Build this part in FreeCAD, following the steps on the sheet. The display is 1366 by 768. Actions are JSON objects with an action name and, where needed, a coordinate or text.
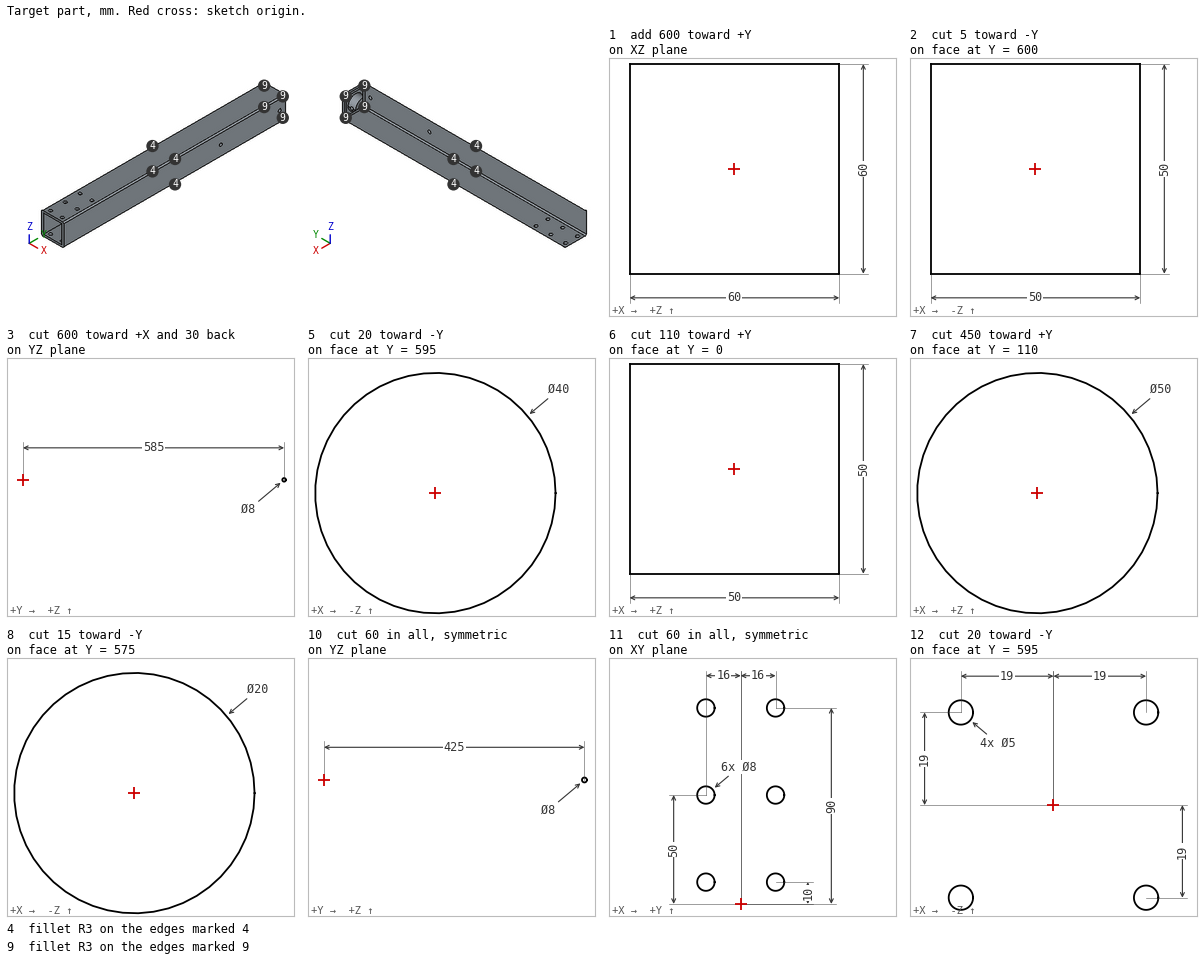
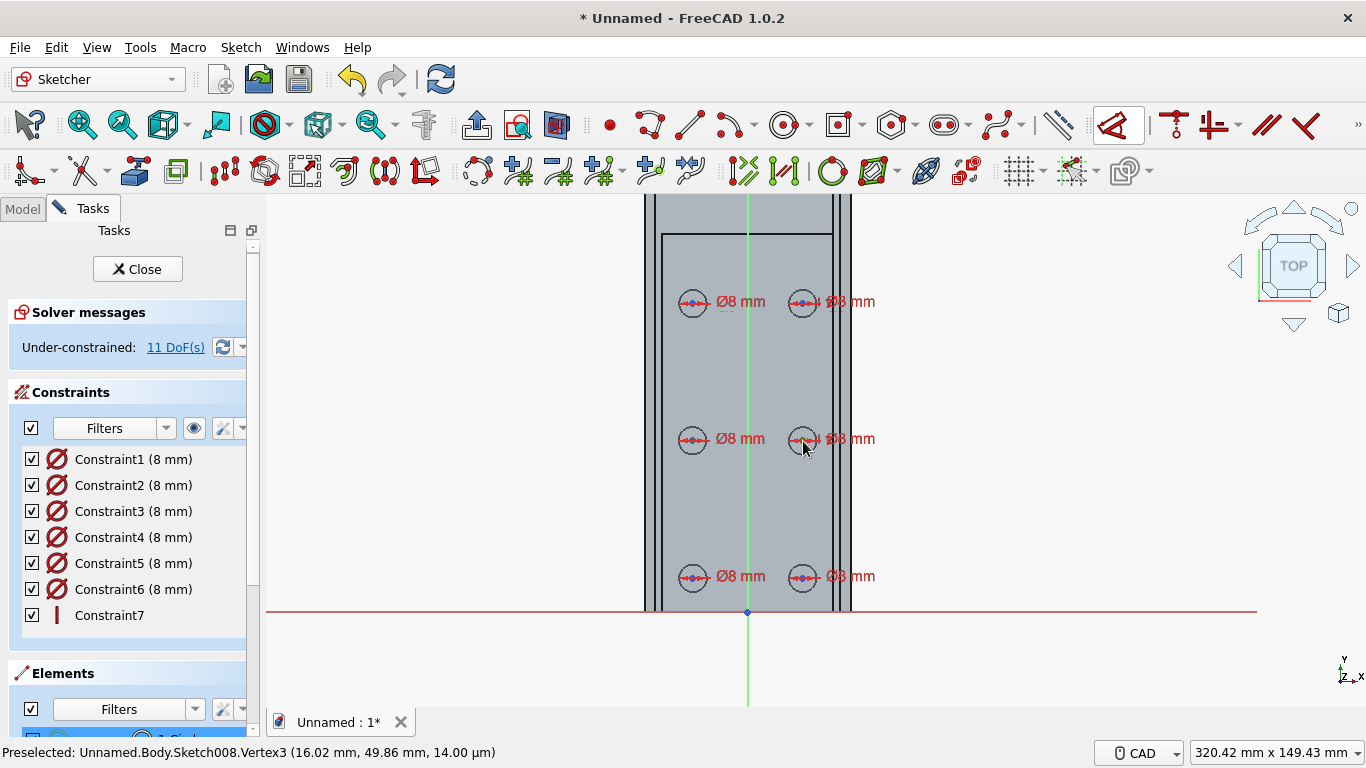
{"action": "key", "text": "h"}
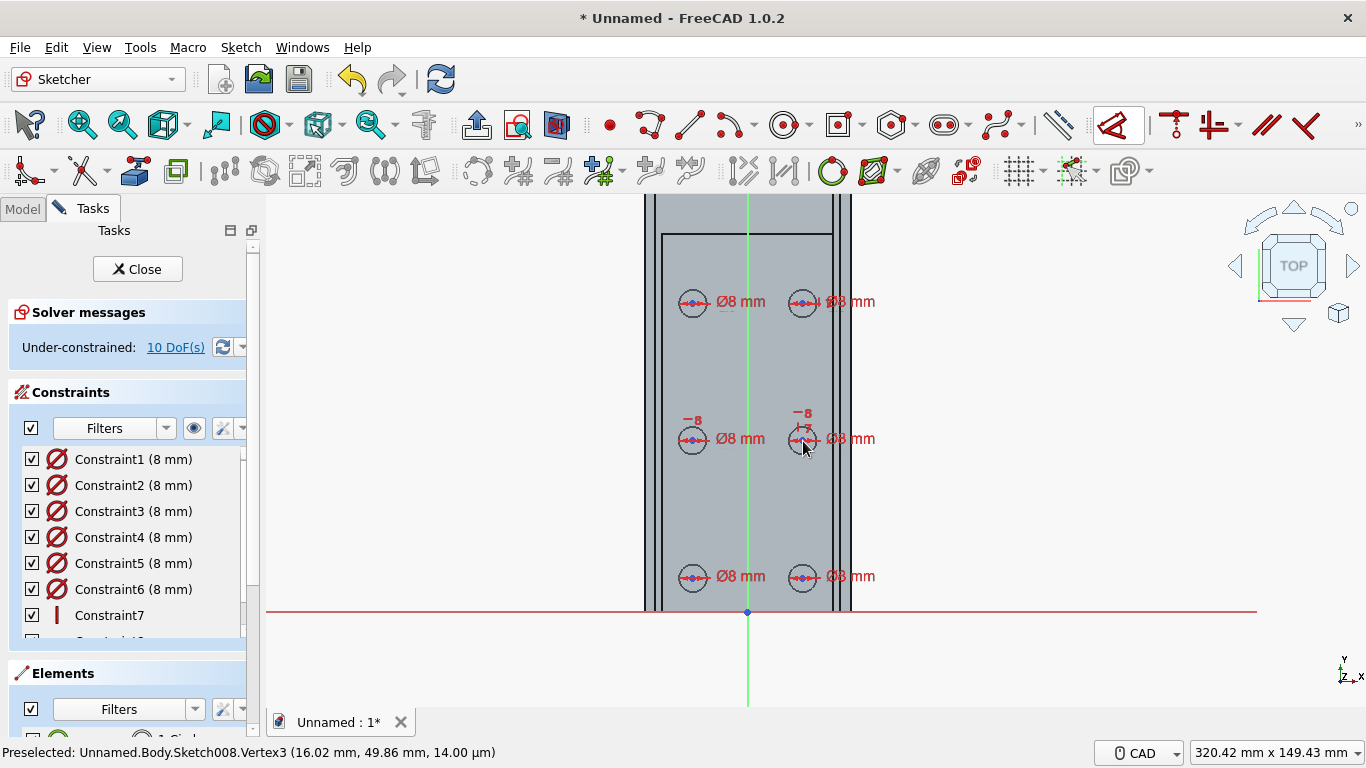
{"action": "left_click", "coordinate": [692, 441]}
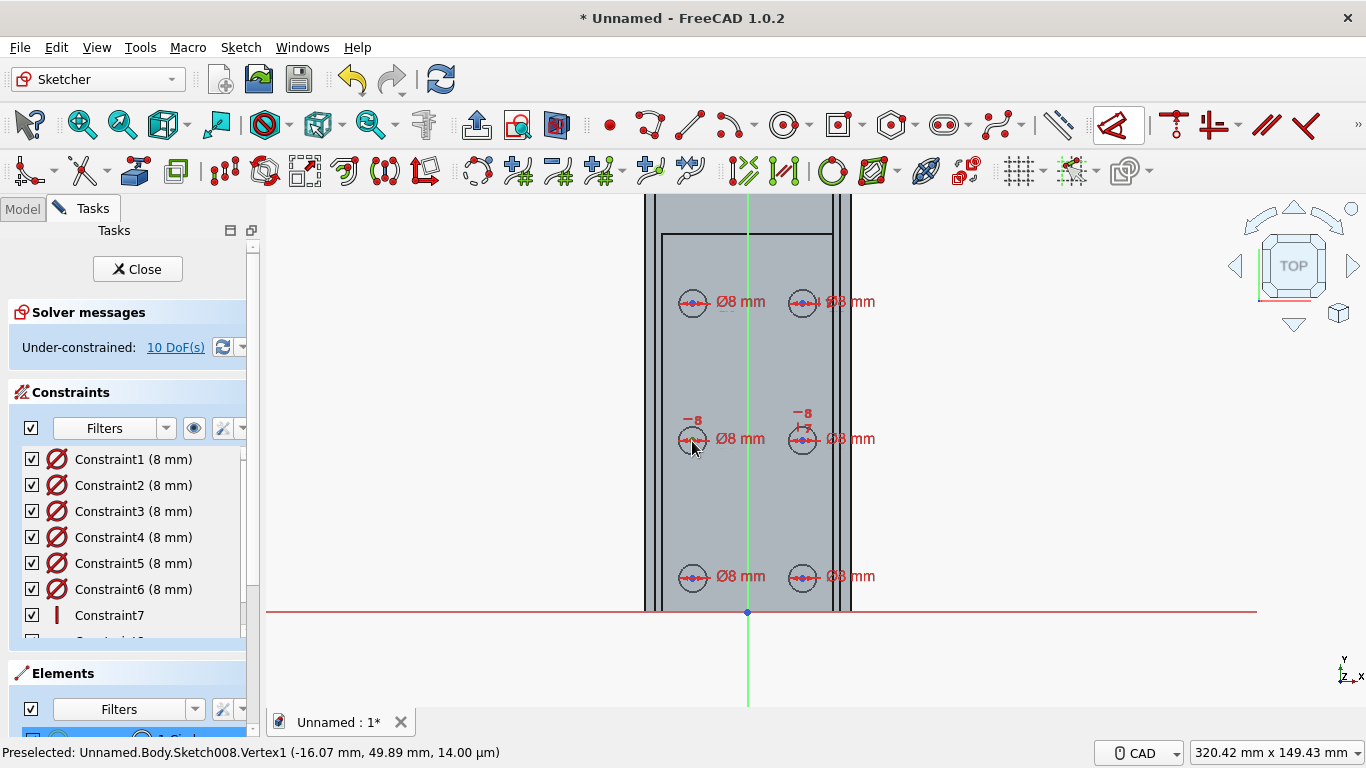
{"action": "left_click", "coordinate": [693, 304]}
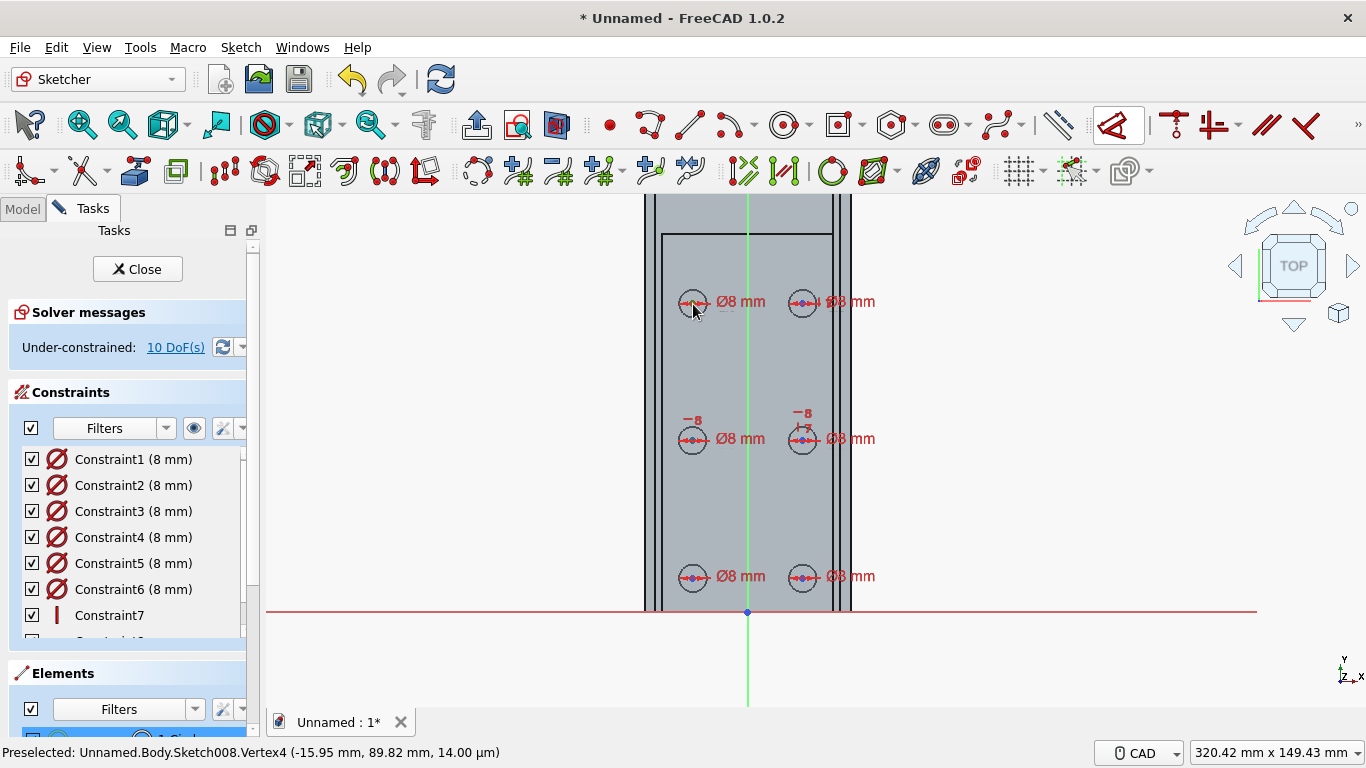
{"action": "left_click", "coordinate": [1240, 126]}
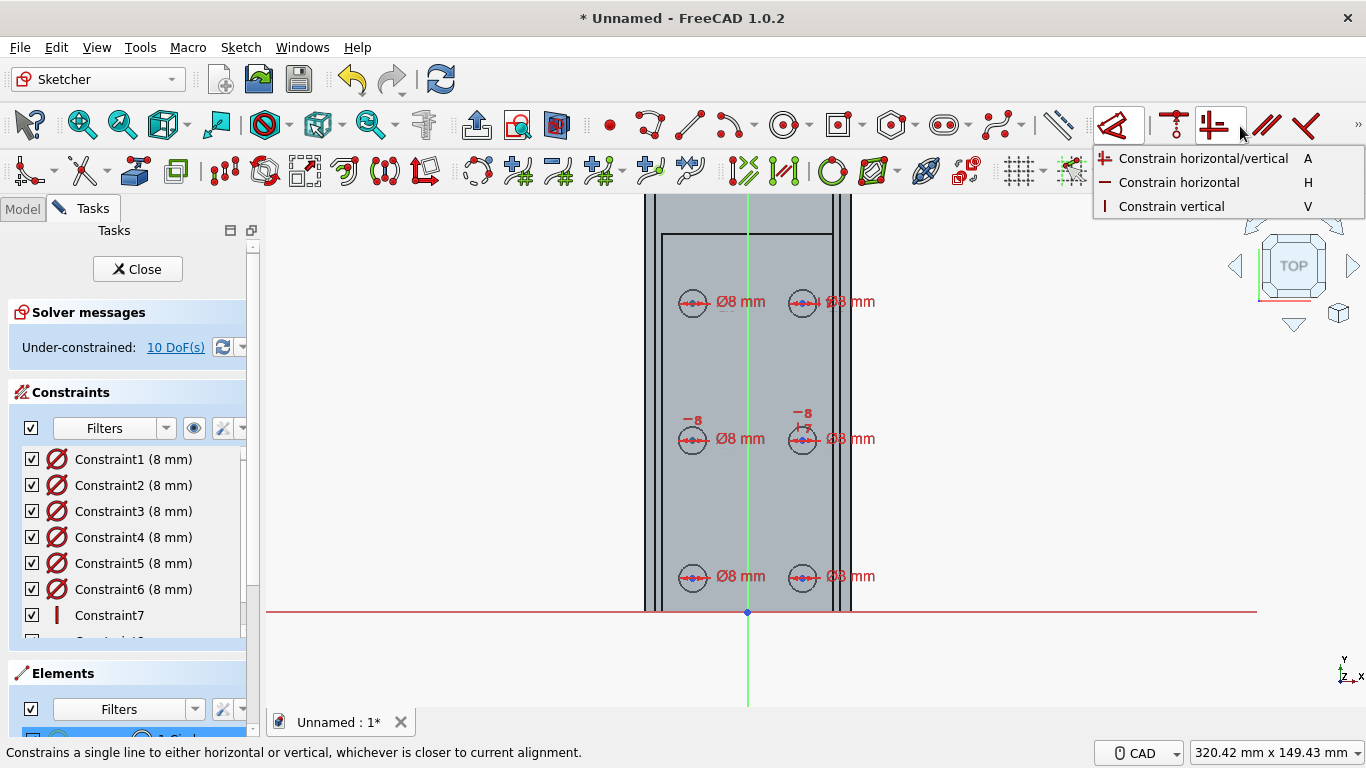
{"action": "left_click", "coordinate": [1229, 206]}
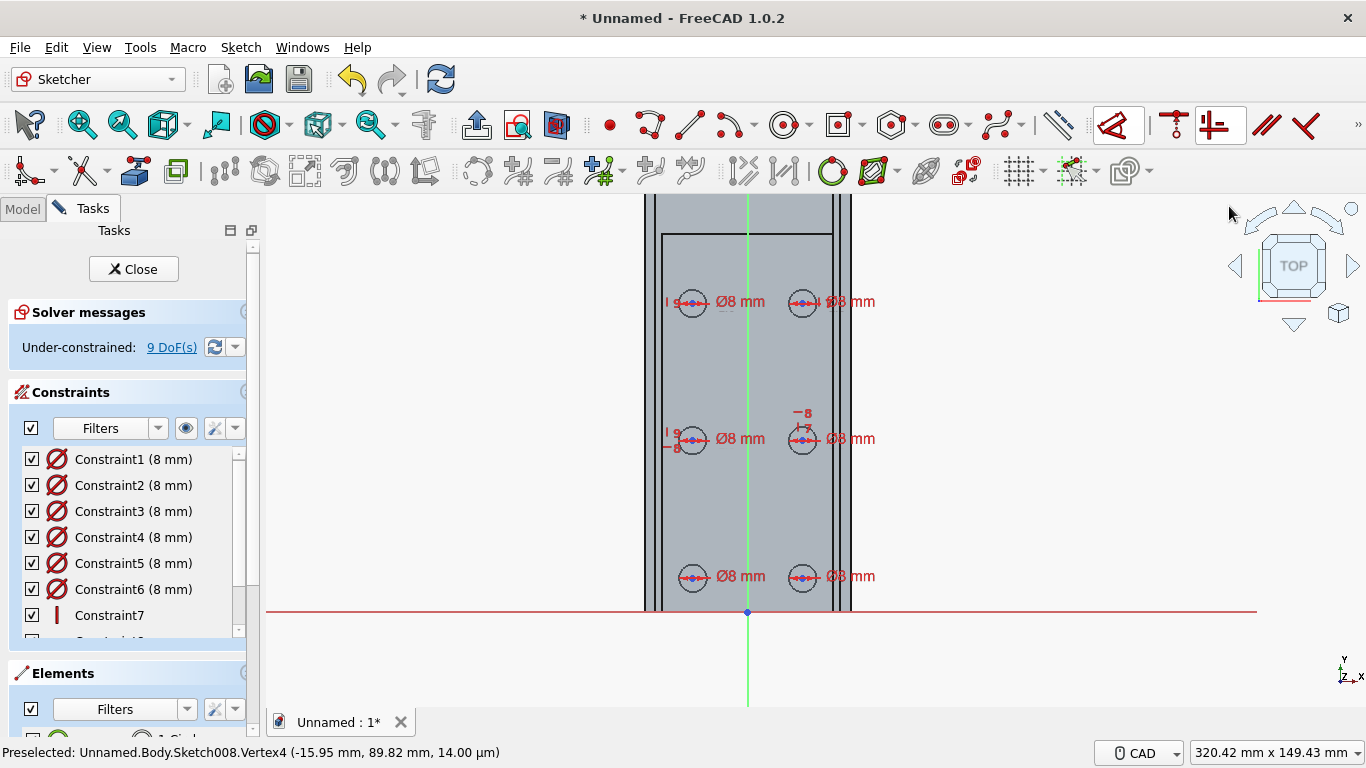
{"action": "left_click", "coordinate": [803, 304]}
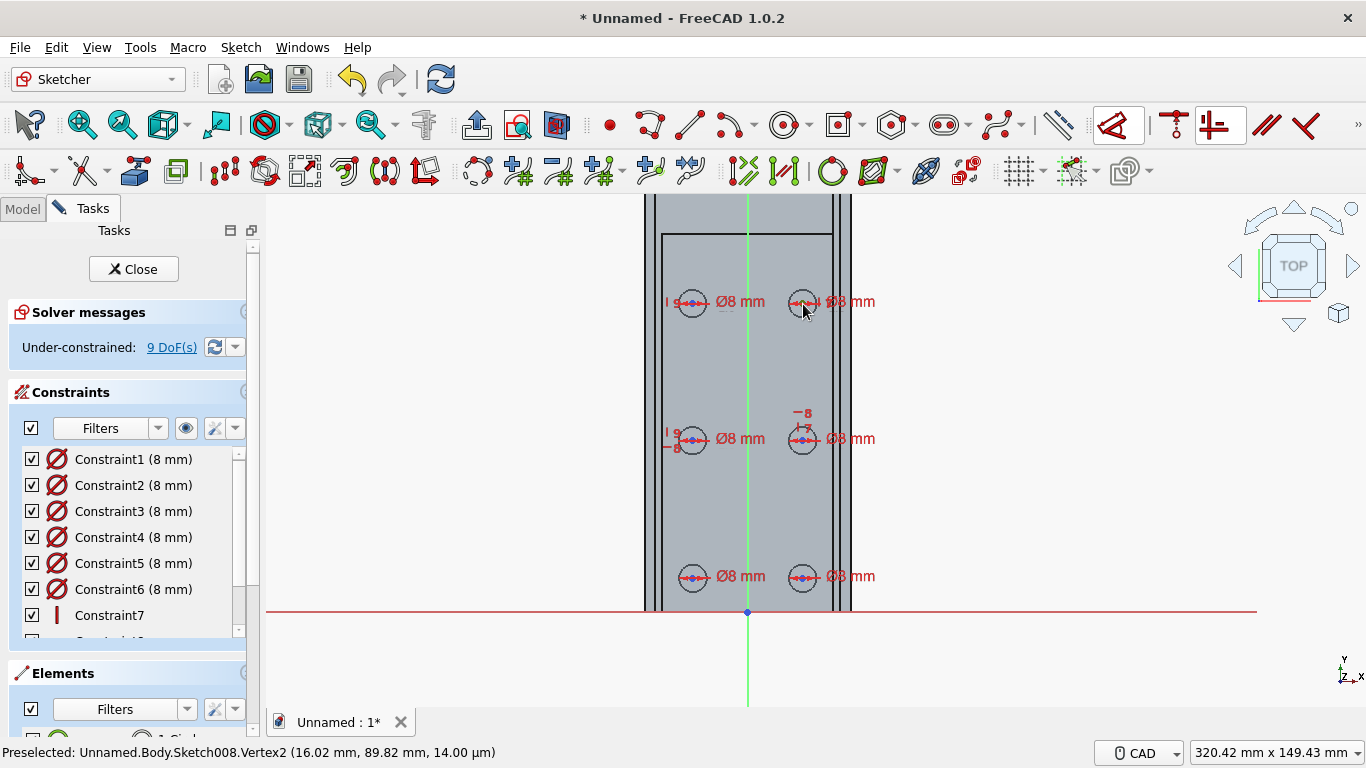
{"action": "left_click", "coordinate": [692, 304]}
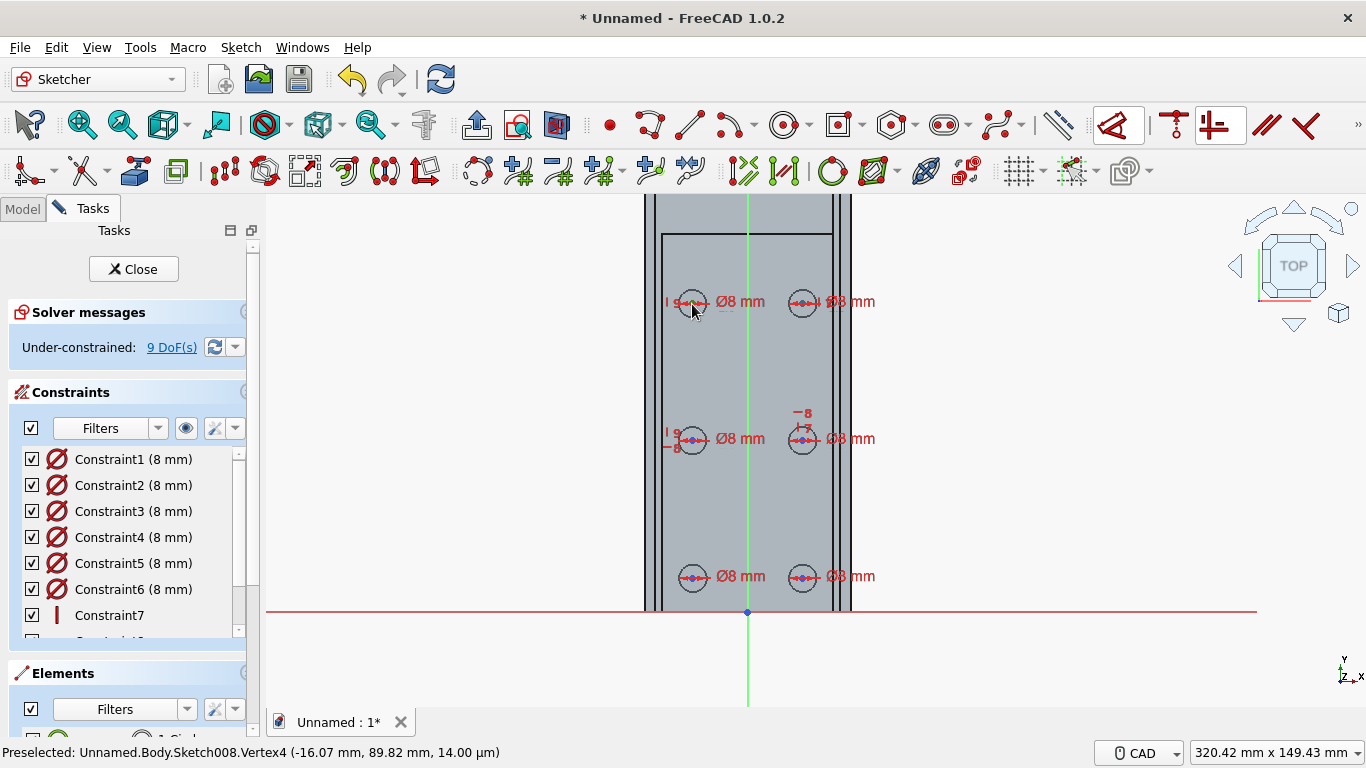
{"action": "key", "text": "h"}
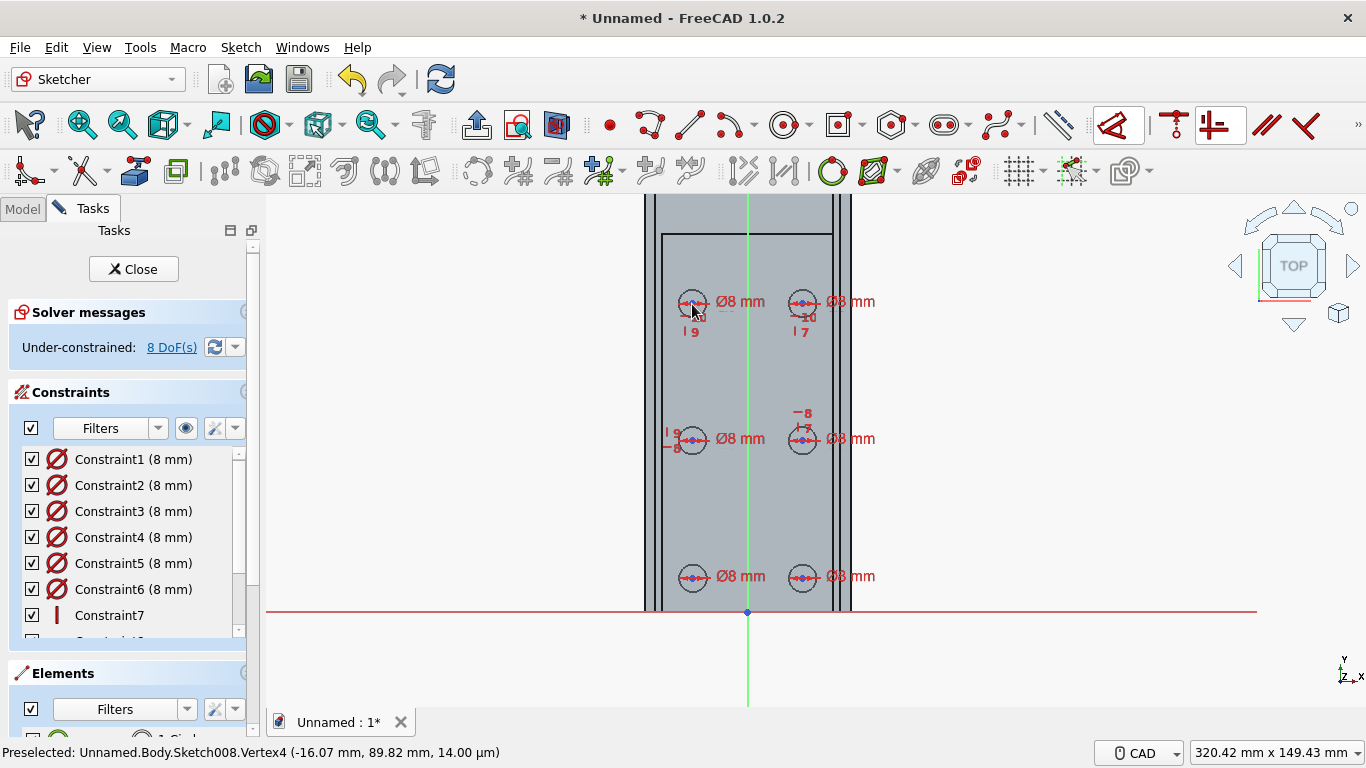
{"action": "left_click", "coordinate": [803, 441]}